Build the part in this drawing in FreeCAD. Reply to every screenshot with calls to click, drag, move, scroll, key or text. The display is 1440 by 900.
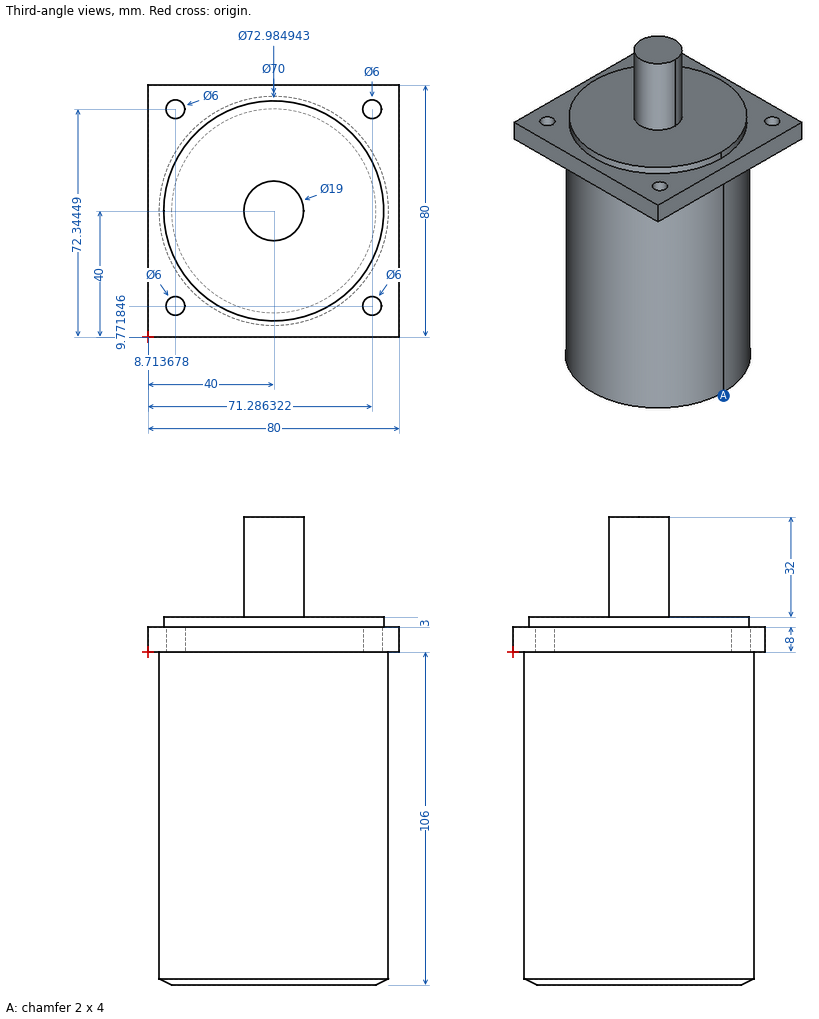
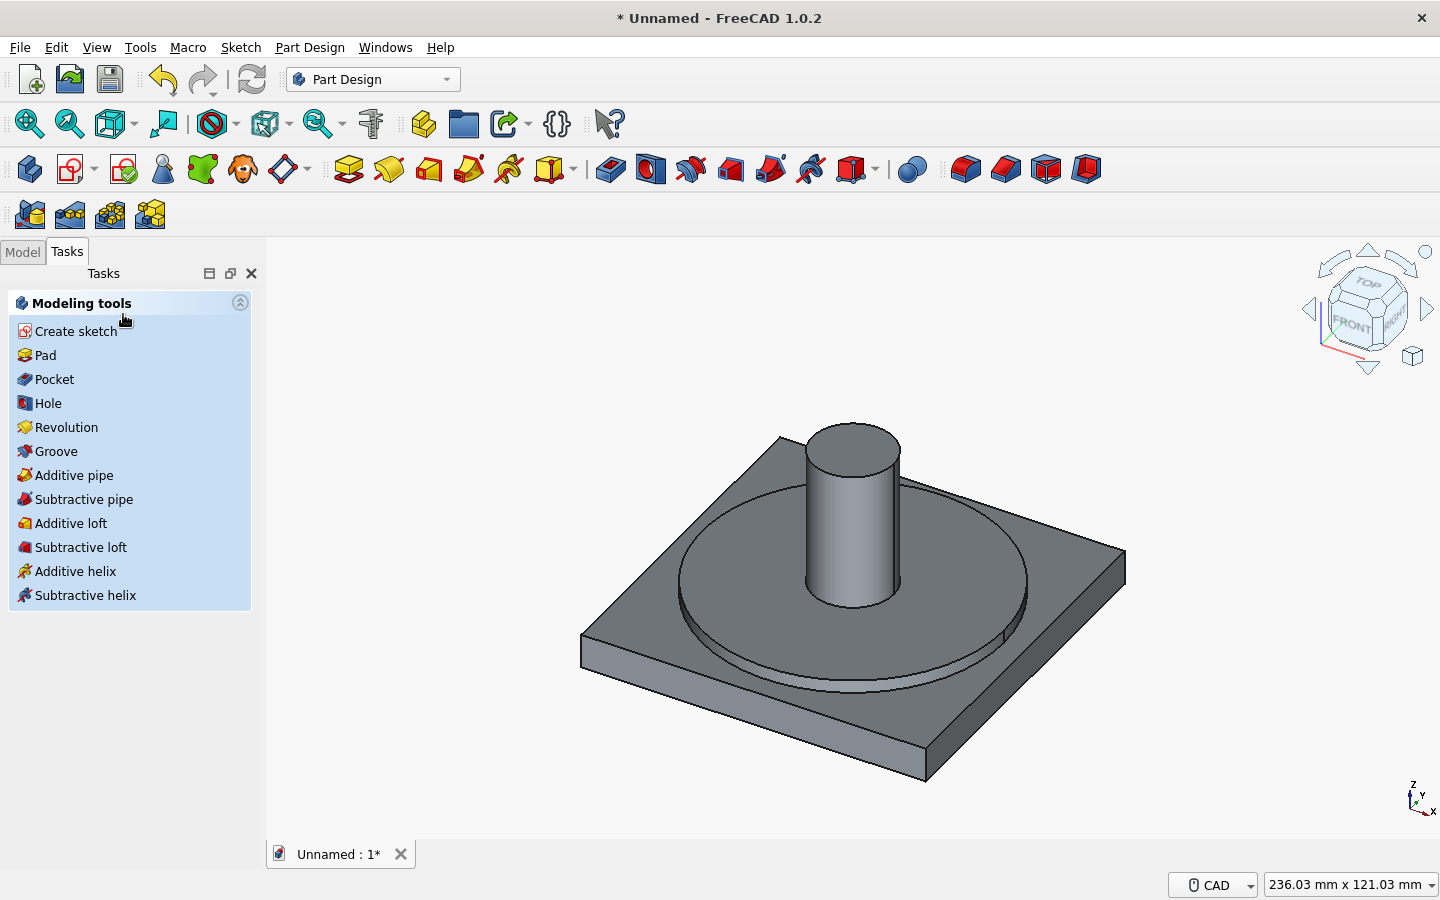
click(350, 170)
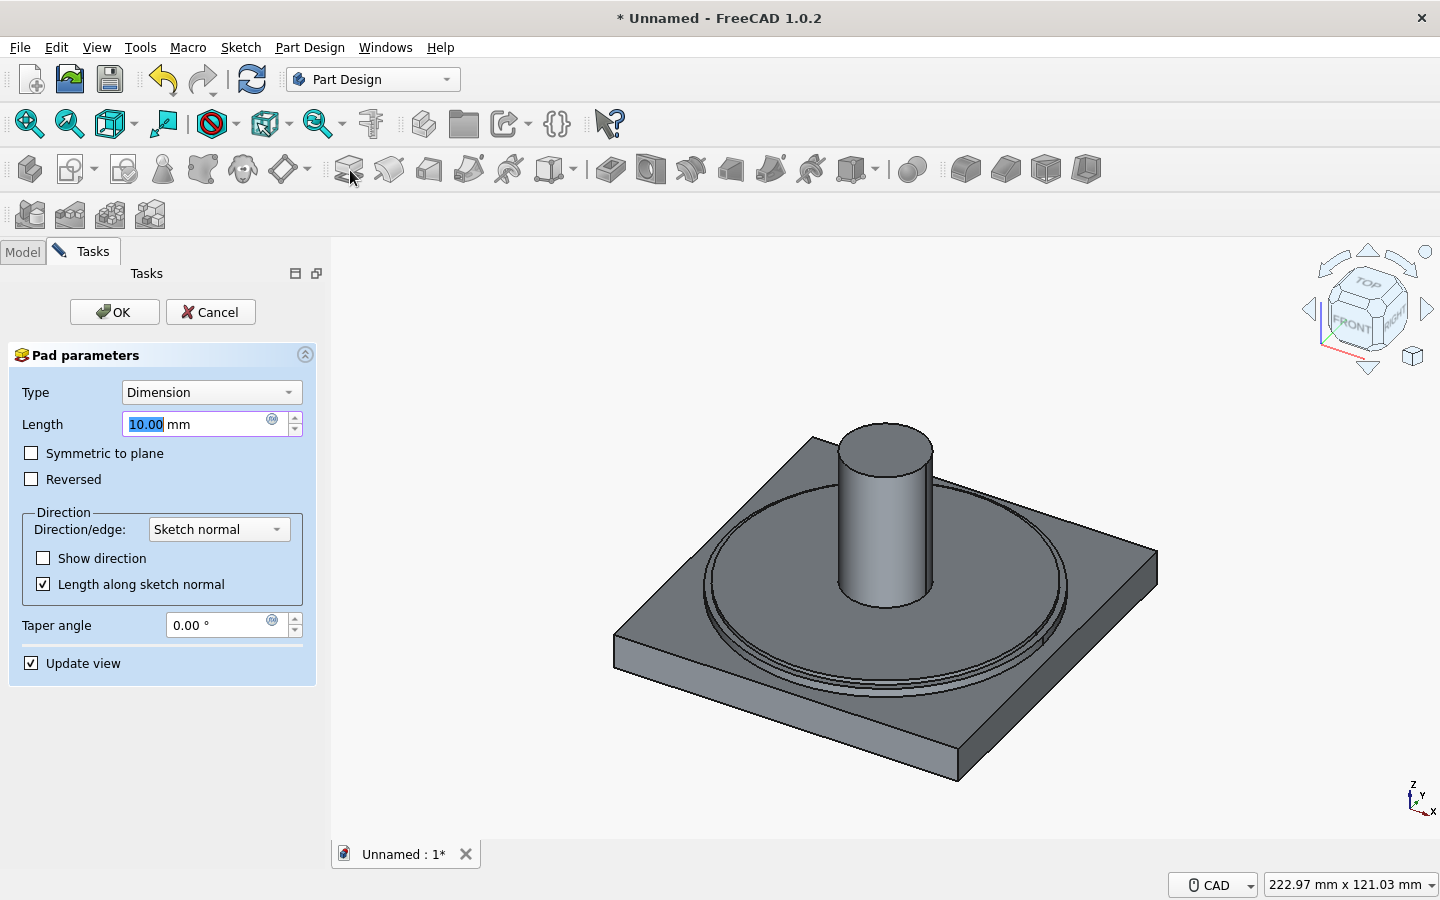
text(106)
key(Tab)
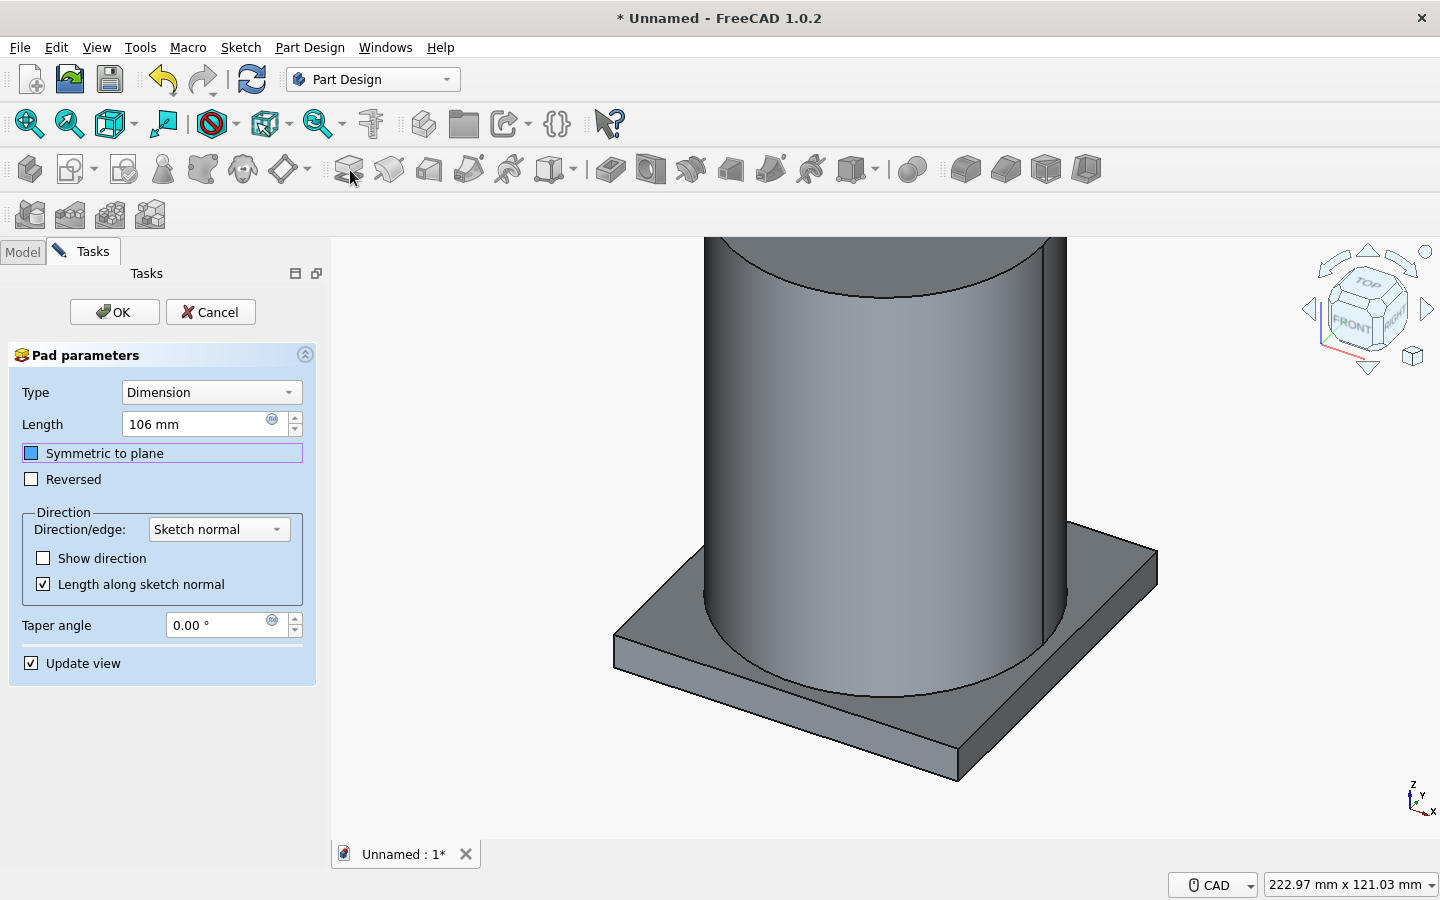
click(30, 479)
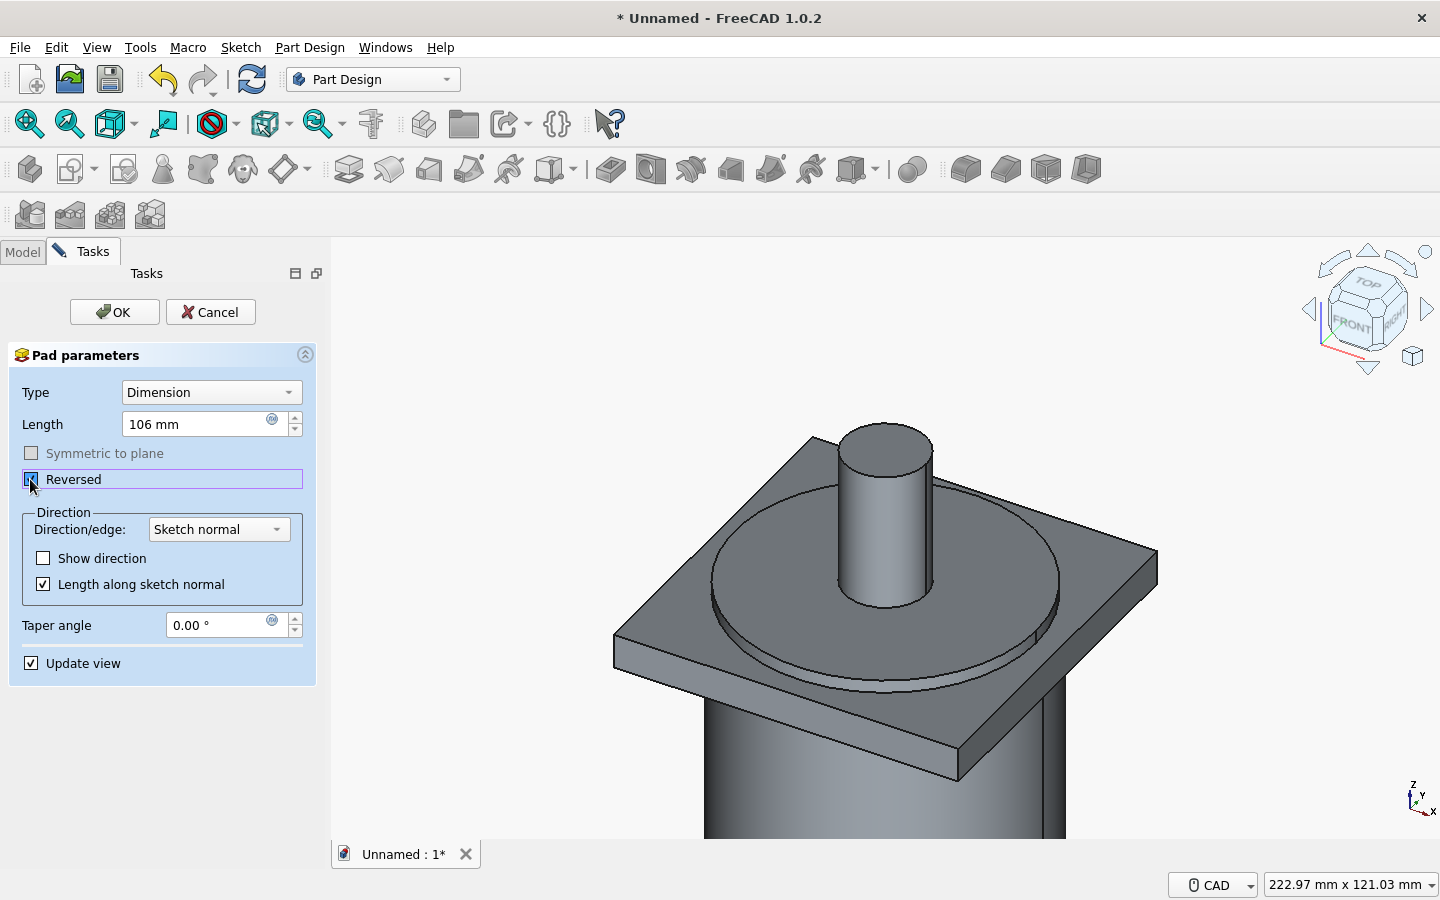
click(115, 312)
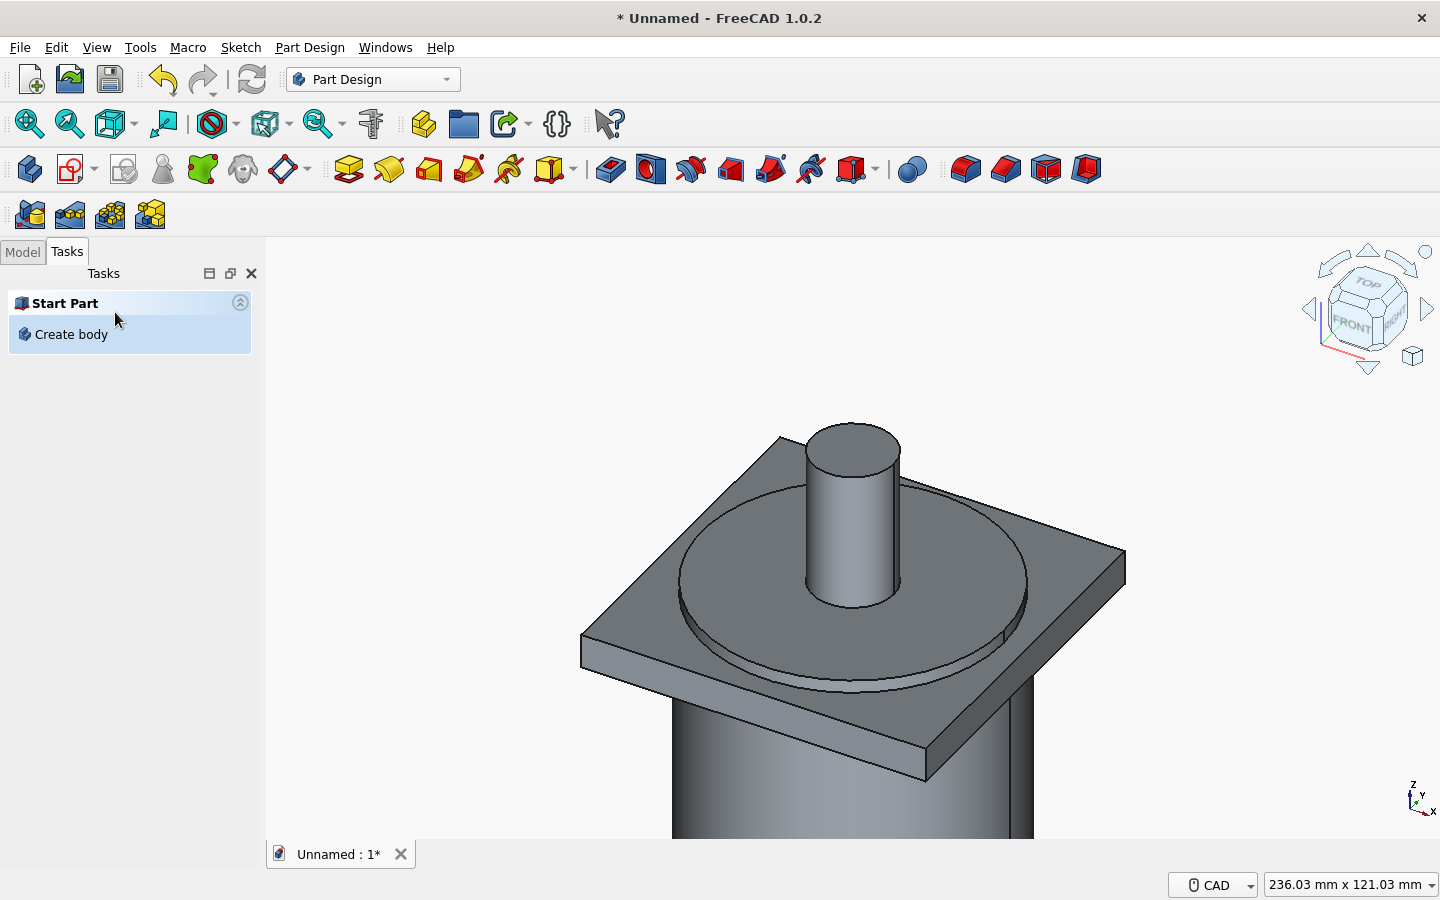
click(30, 124)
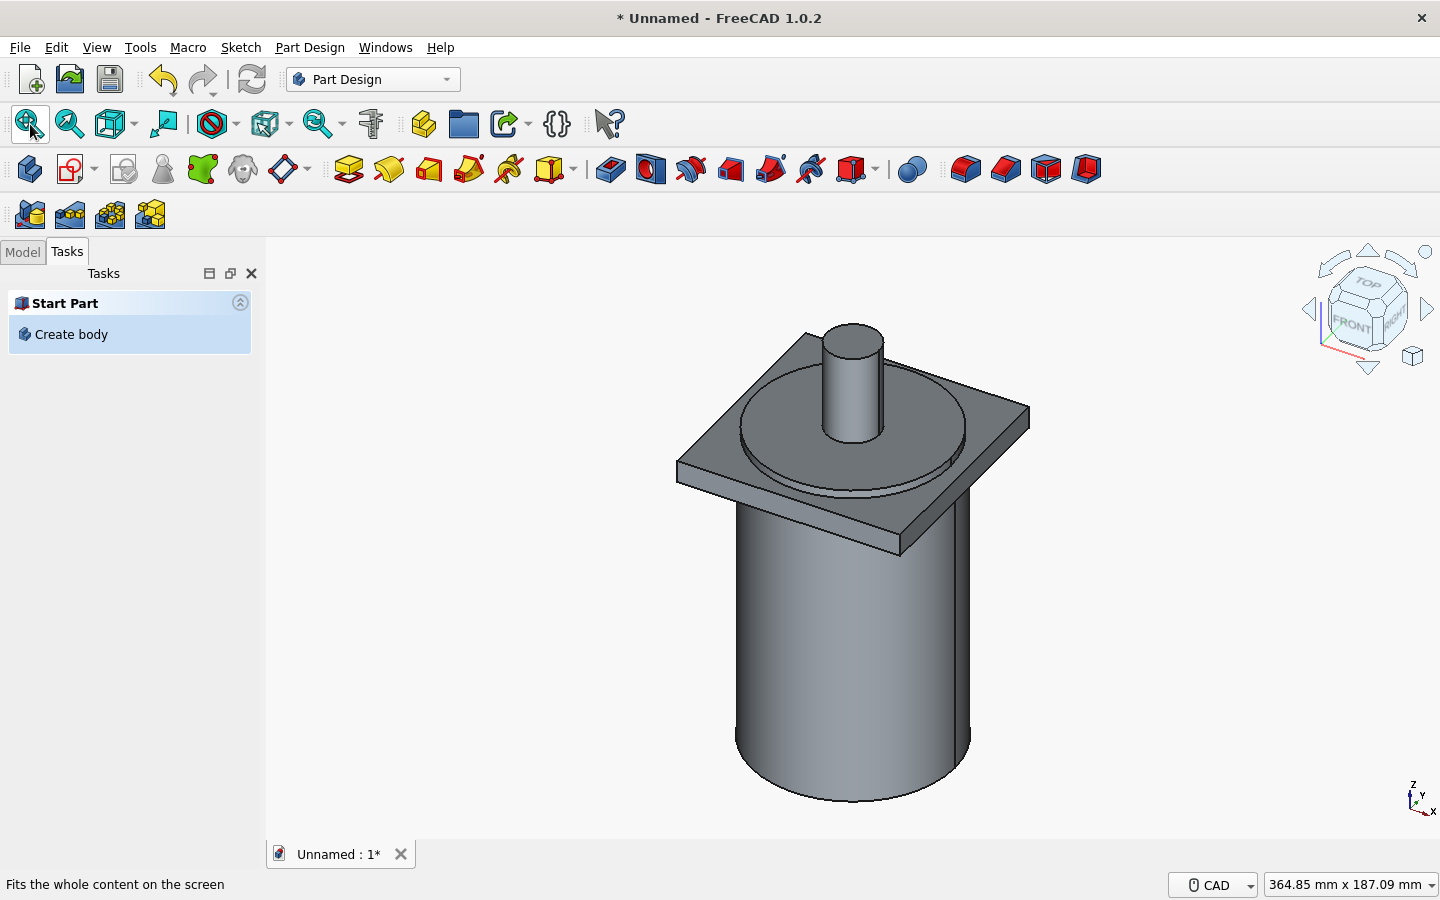
click(862, 509)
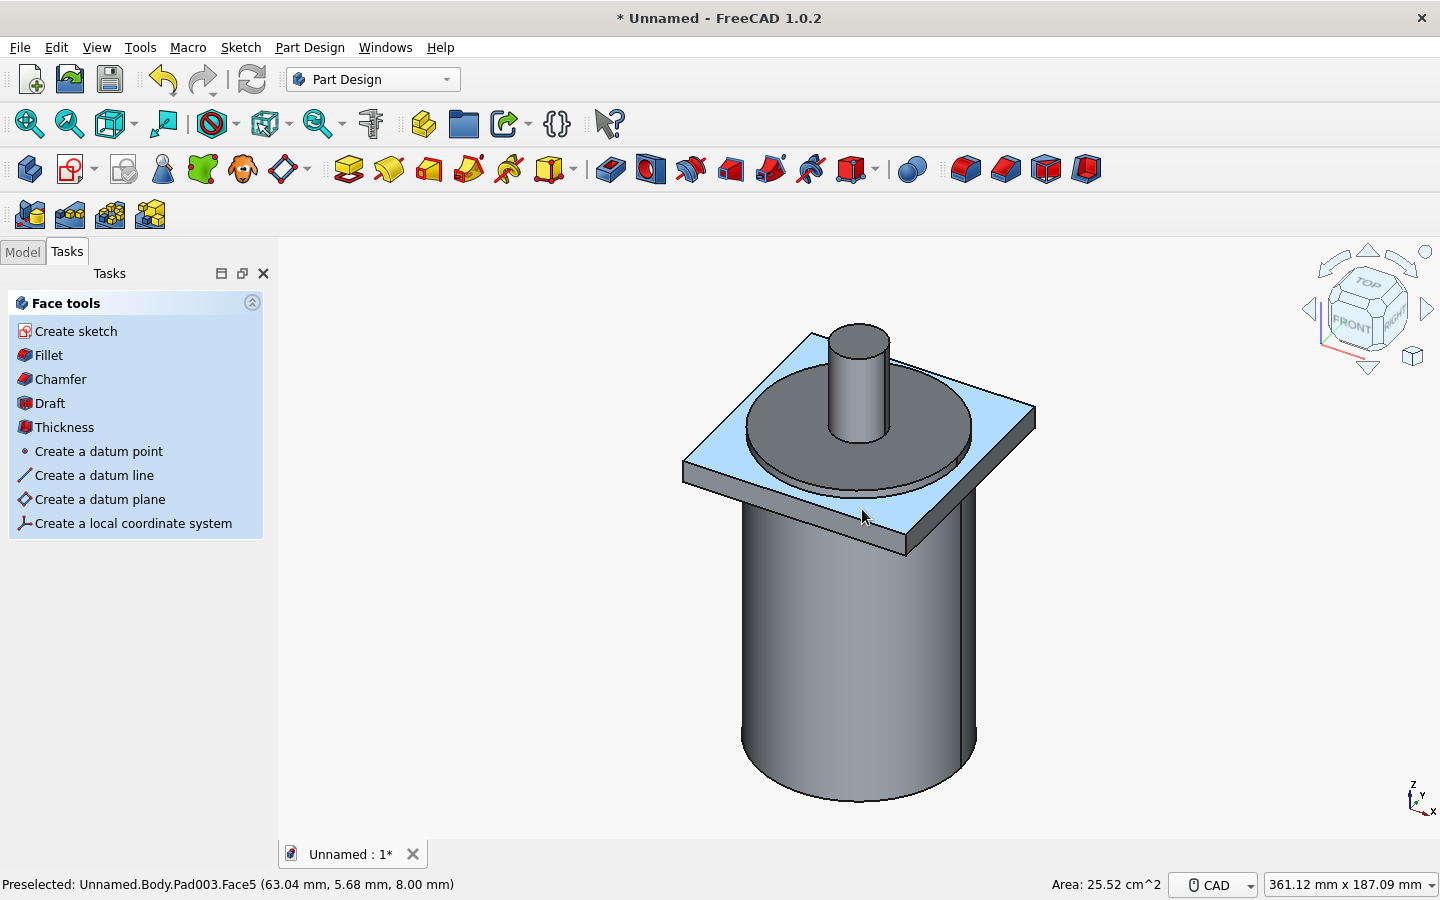
click(70, 170)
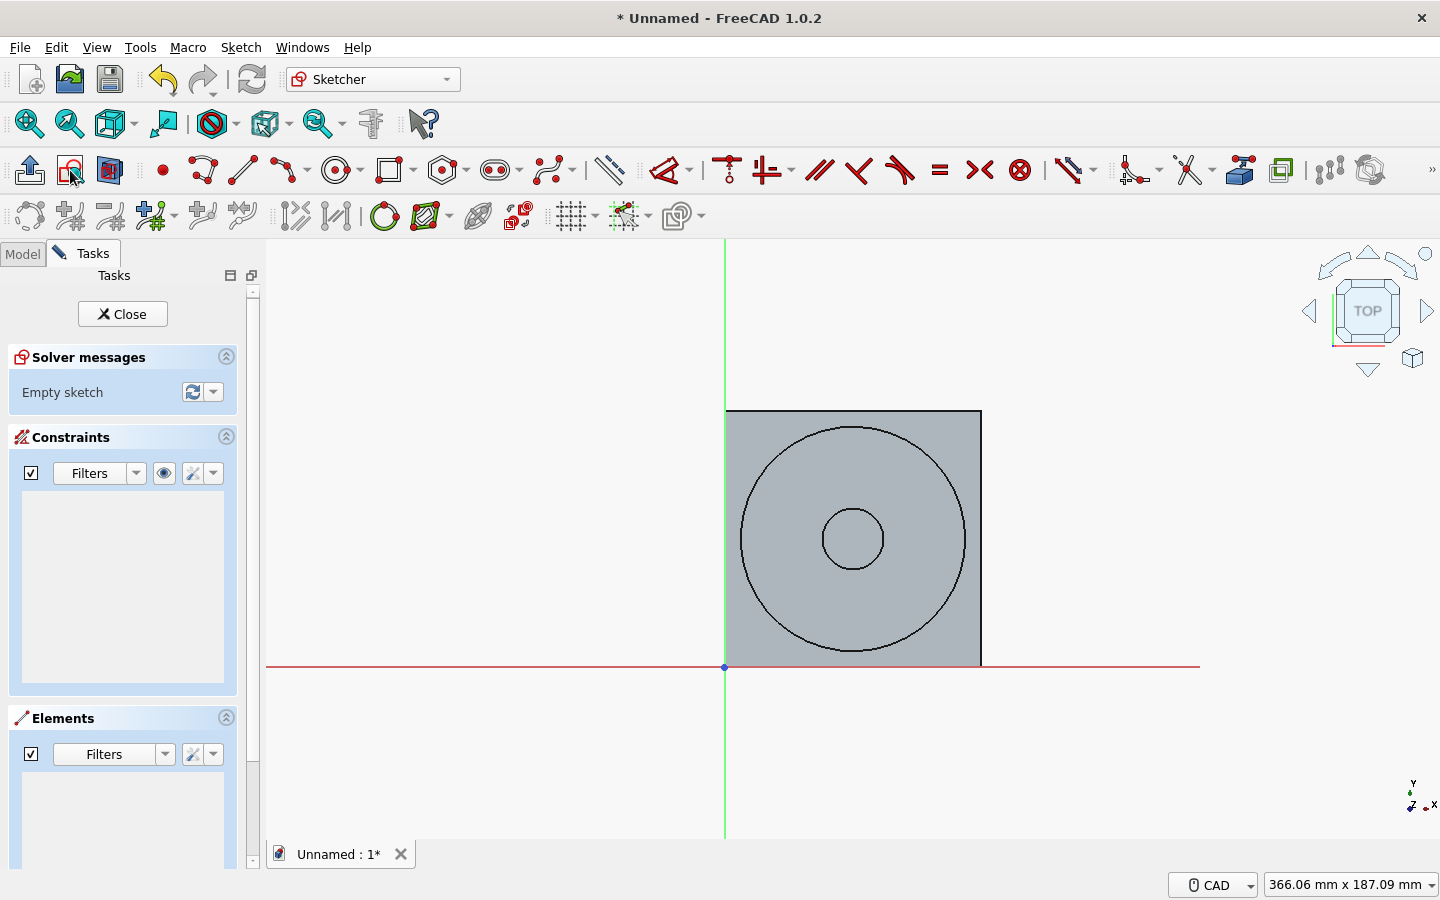
scroll(751, 430, up, 15)